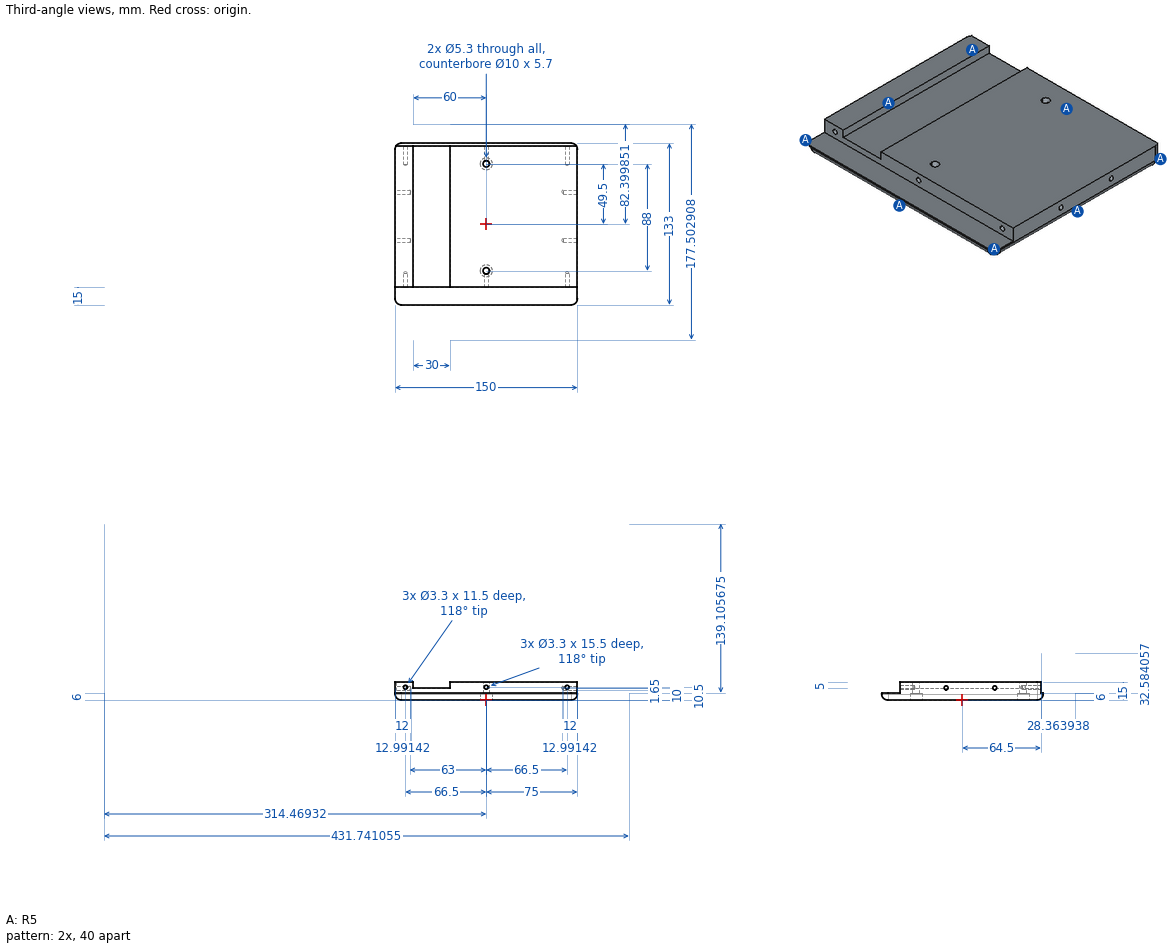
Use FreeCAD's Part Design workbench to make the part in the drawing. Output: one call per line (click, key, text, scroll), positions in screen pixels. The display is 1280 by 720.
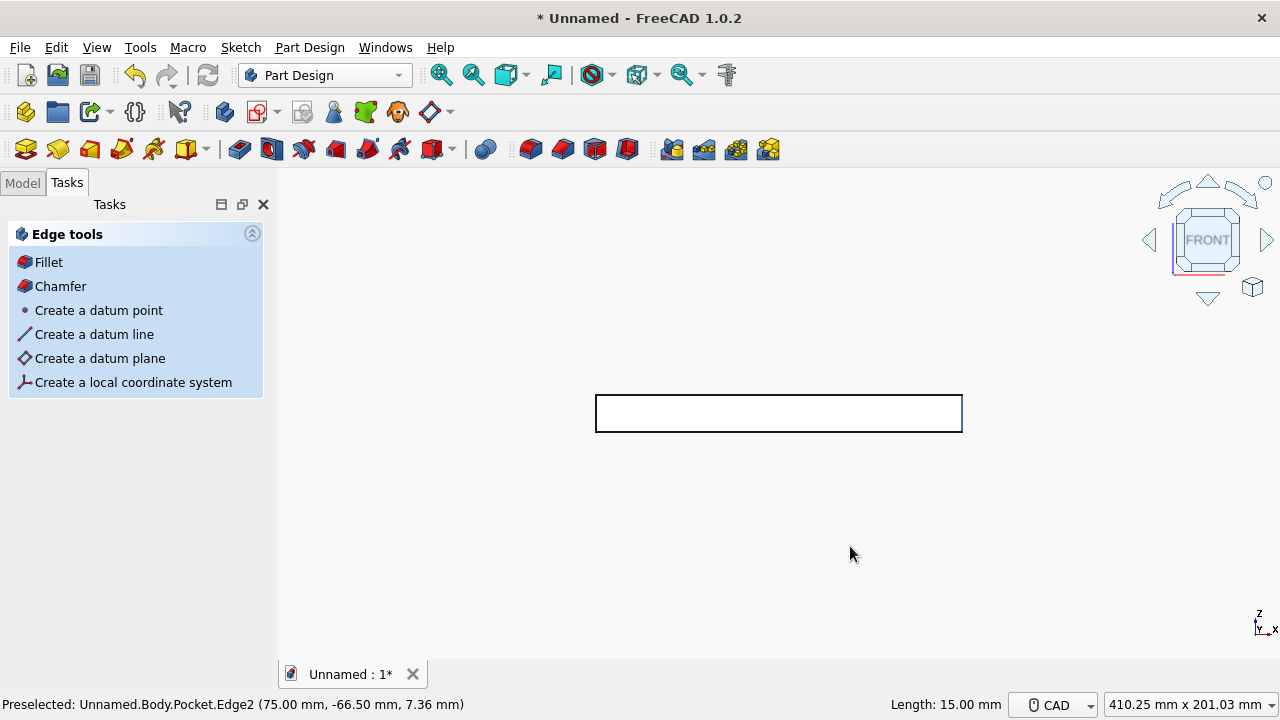
click(442, 76)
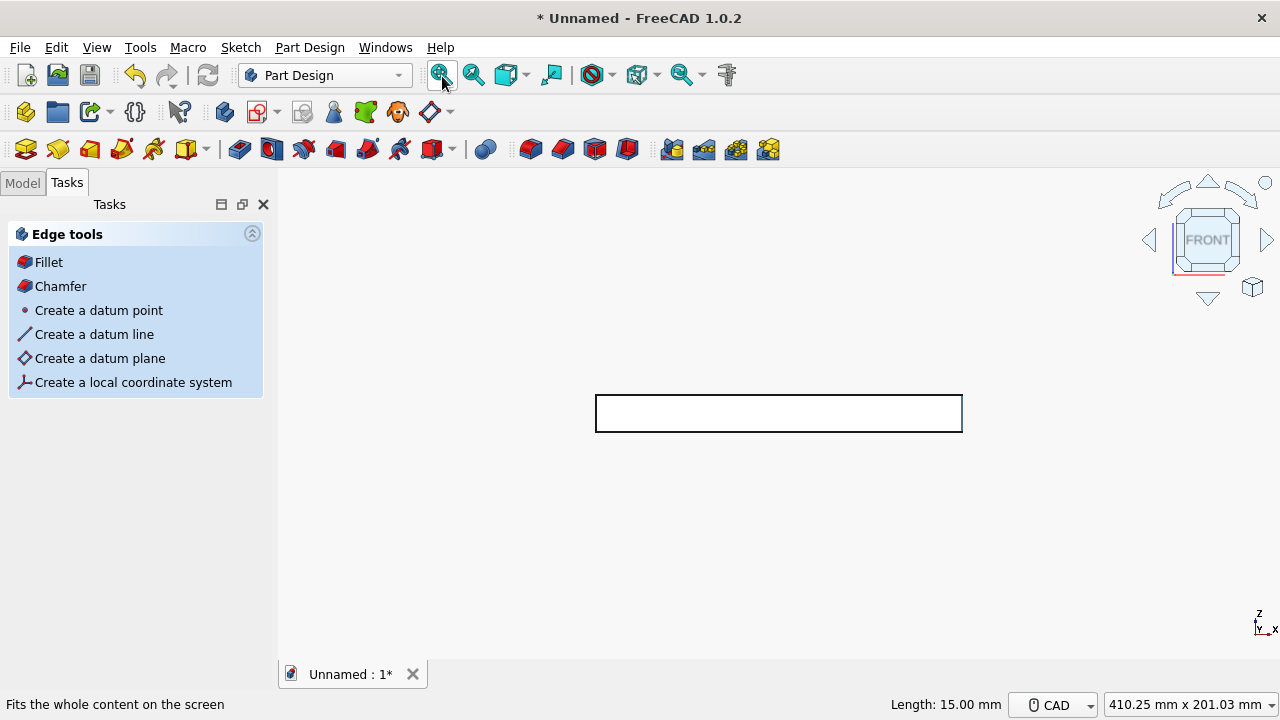
click(596, 413, ctrl)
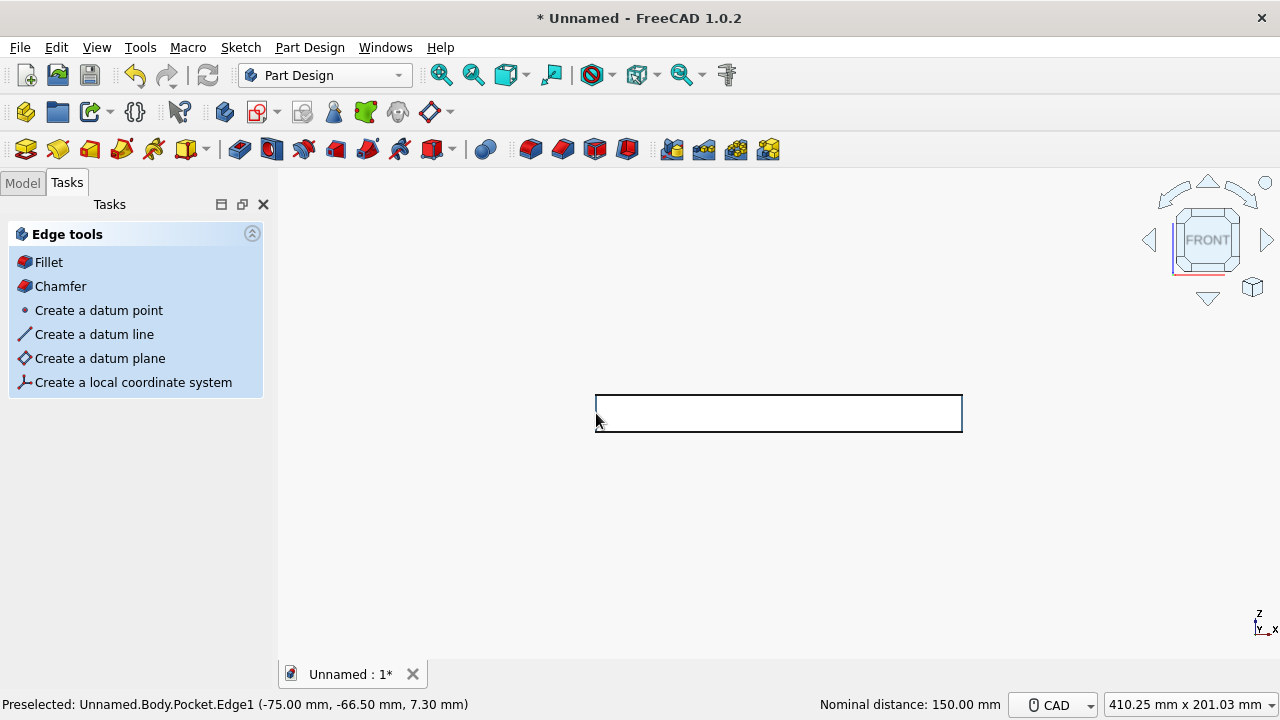
key(3)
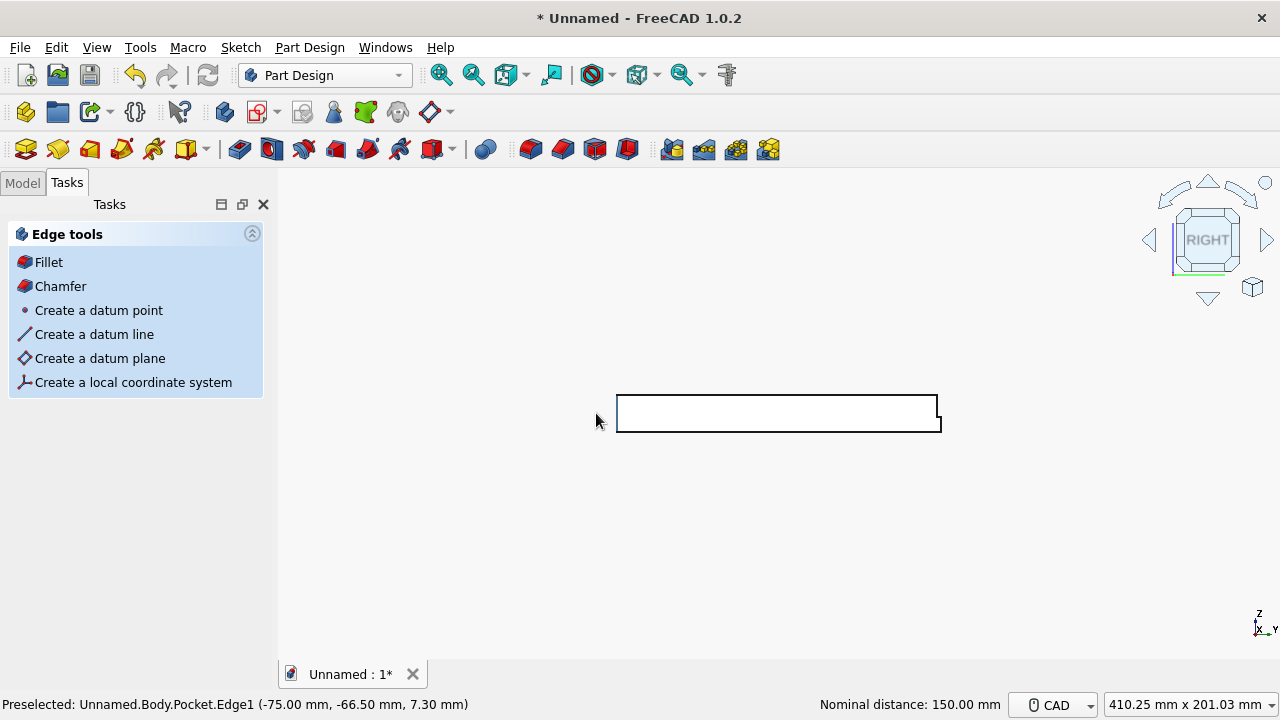
click(442, 76)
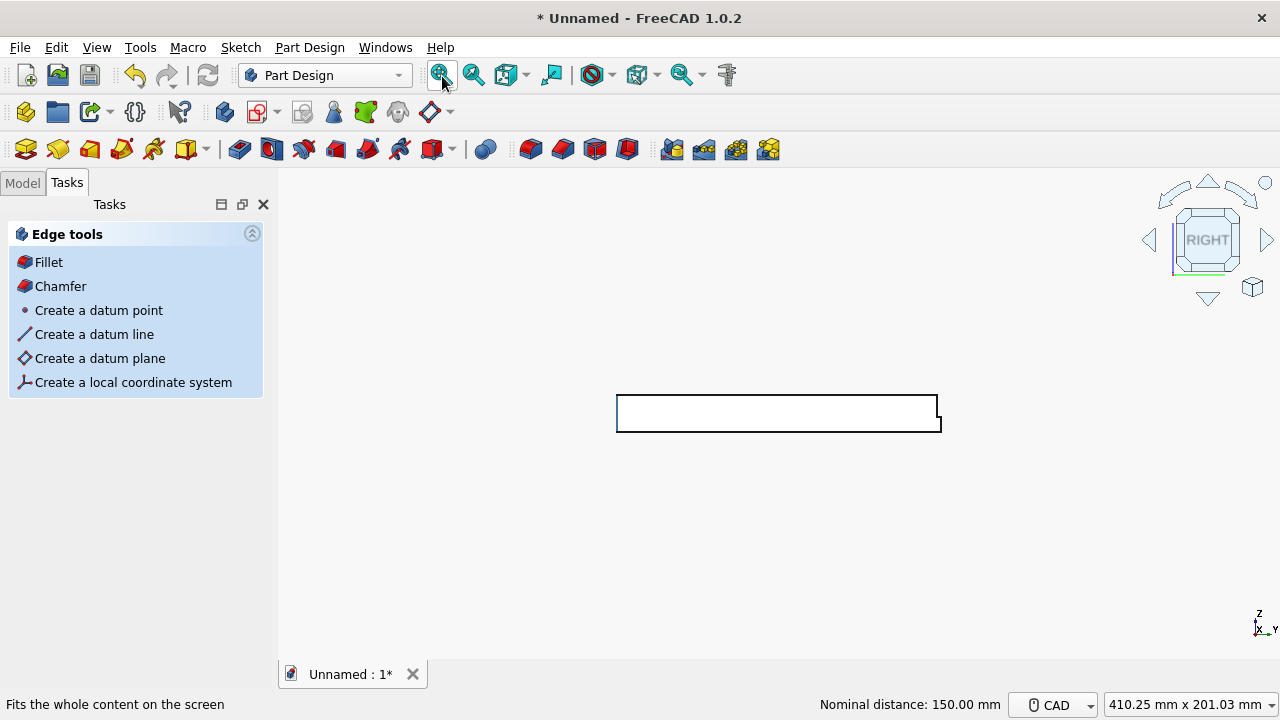
click(941, 423, ctrl)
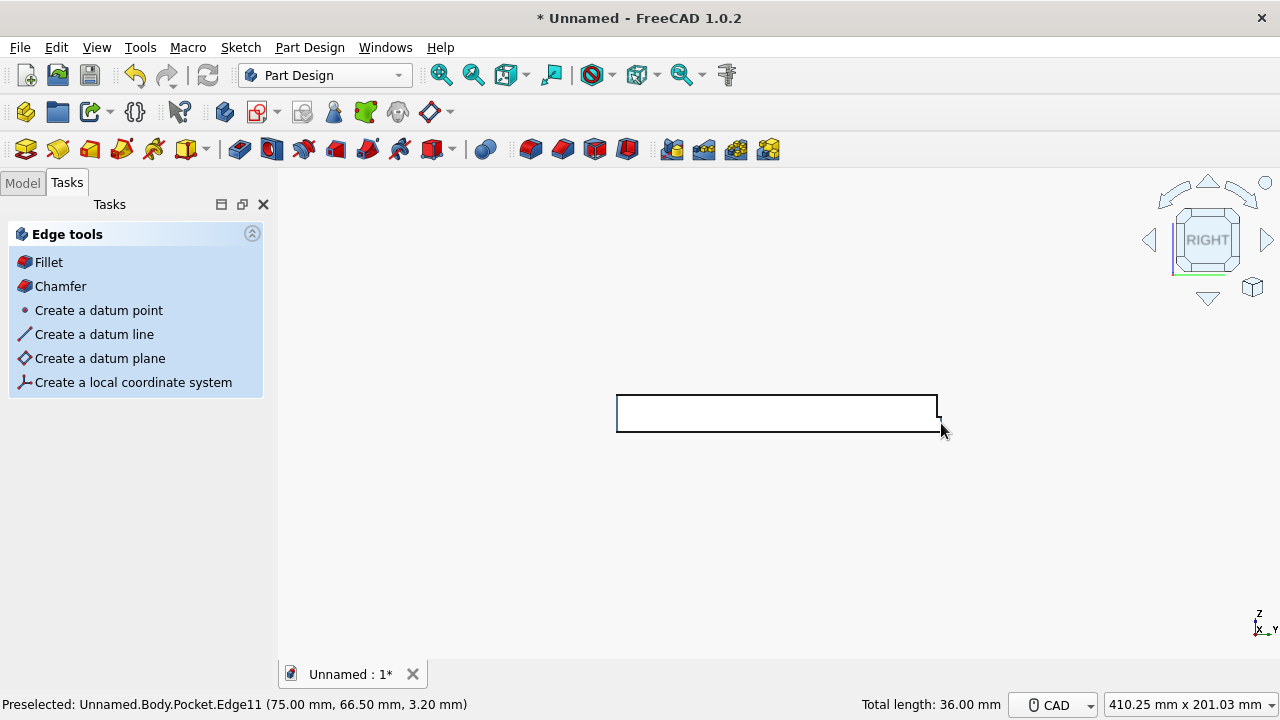
key(5)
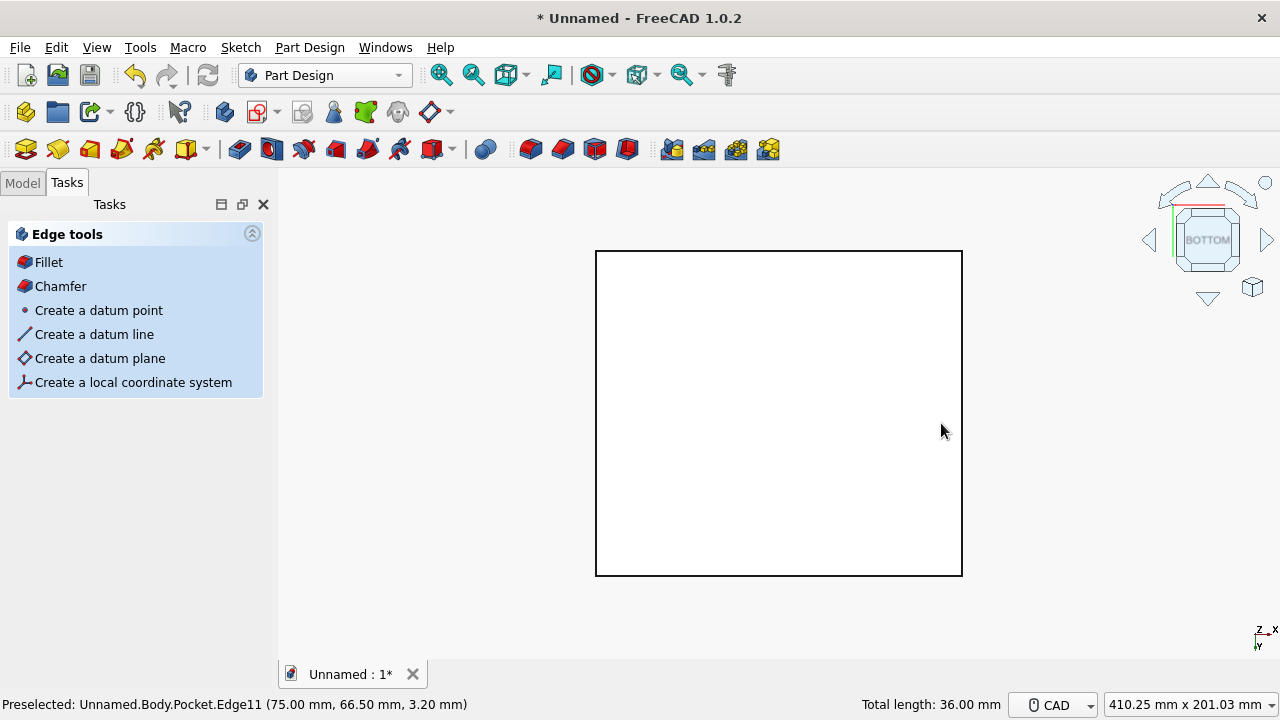
click(779, 412, ctrl)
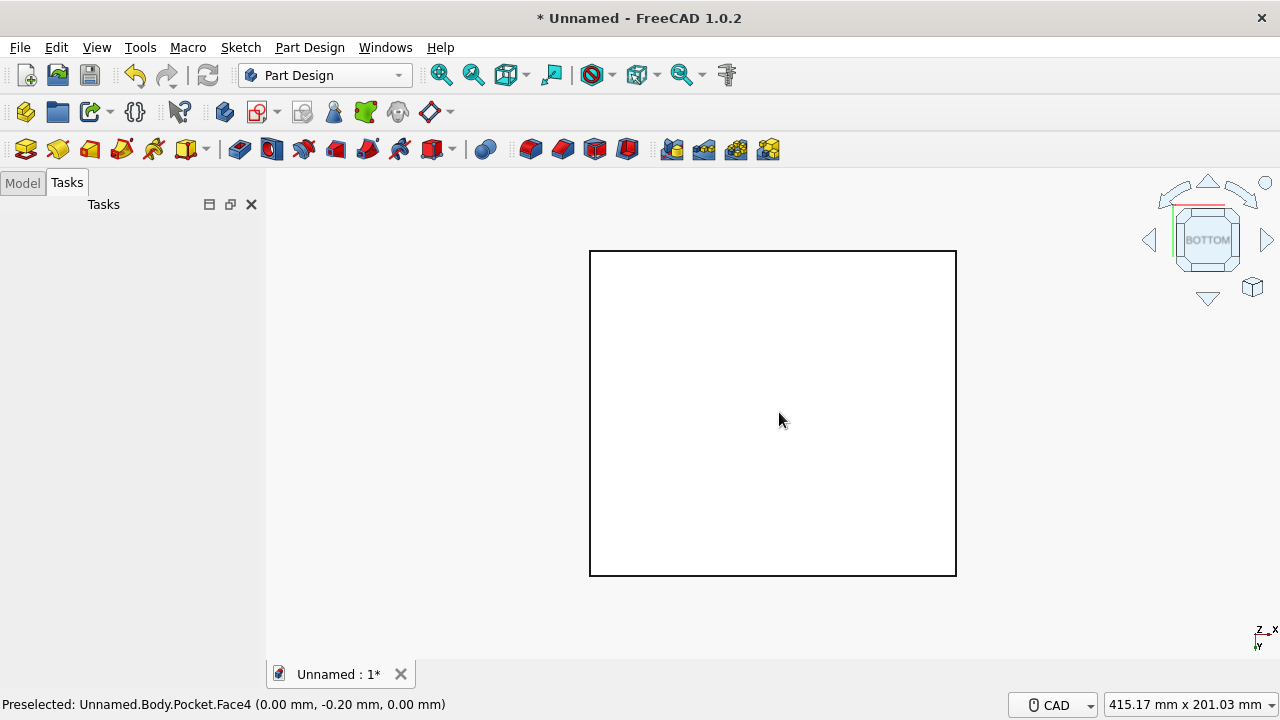
scroll(590, 575, up, 6)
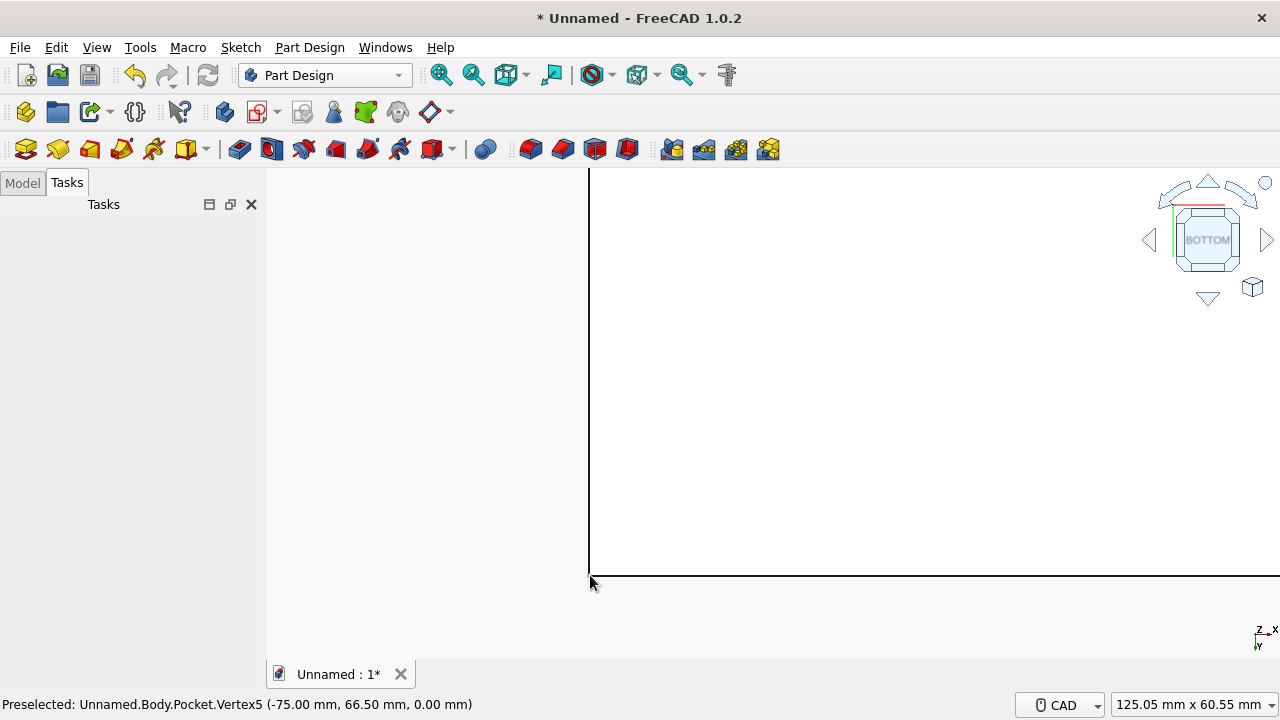
click(442, 76)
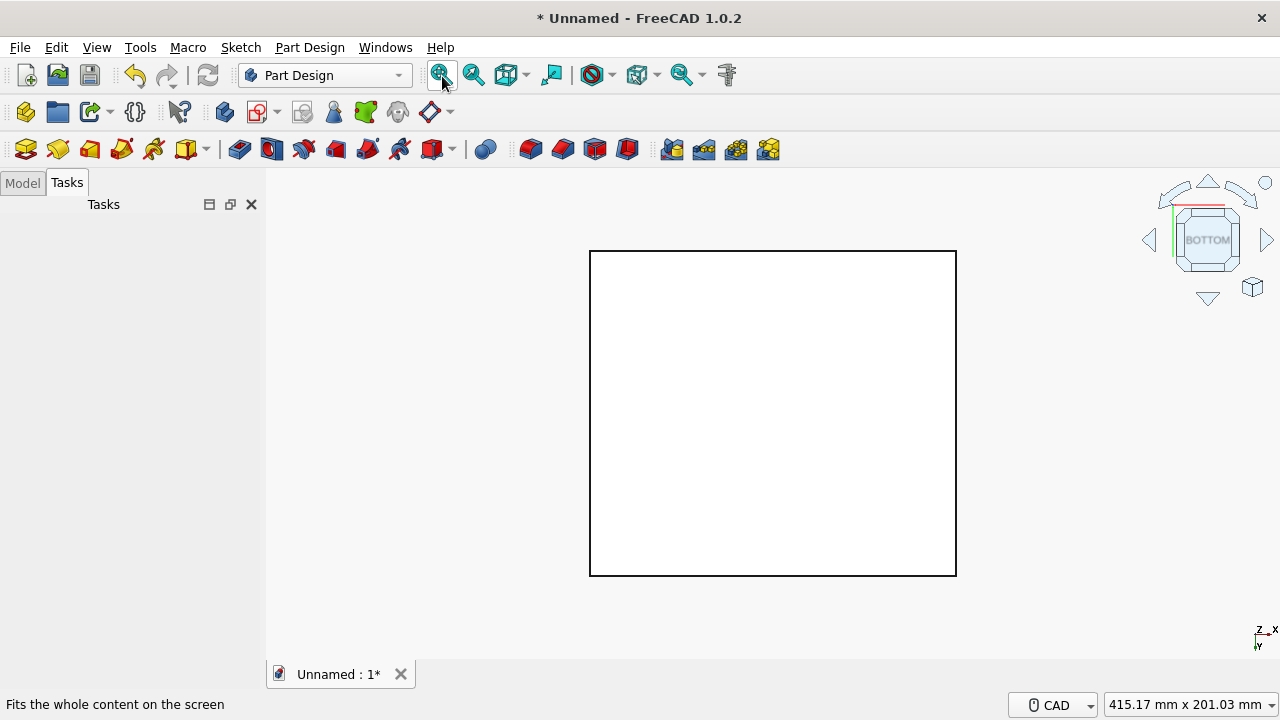
key(4)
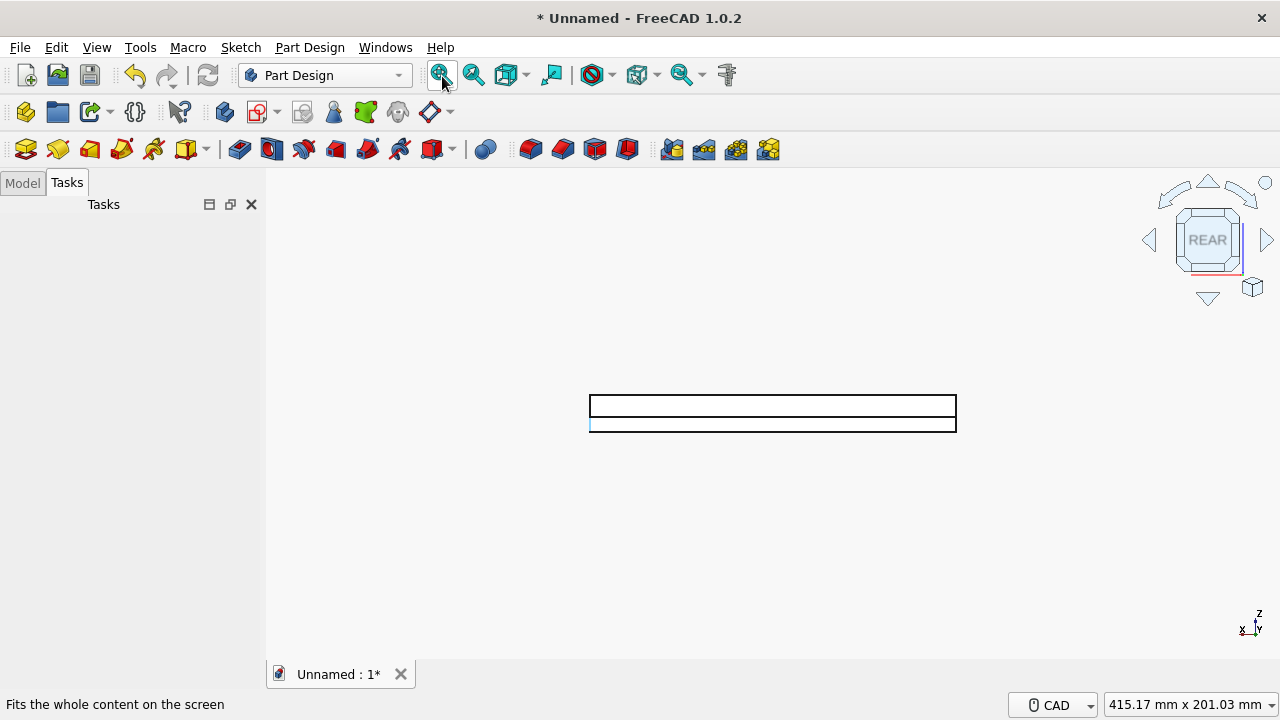
click(442, 76)